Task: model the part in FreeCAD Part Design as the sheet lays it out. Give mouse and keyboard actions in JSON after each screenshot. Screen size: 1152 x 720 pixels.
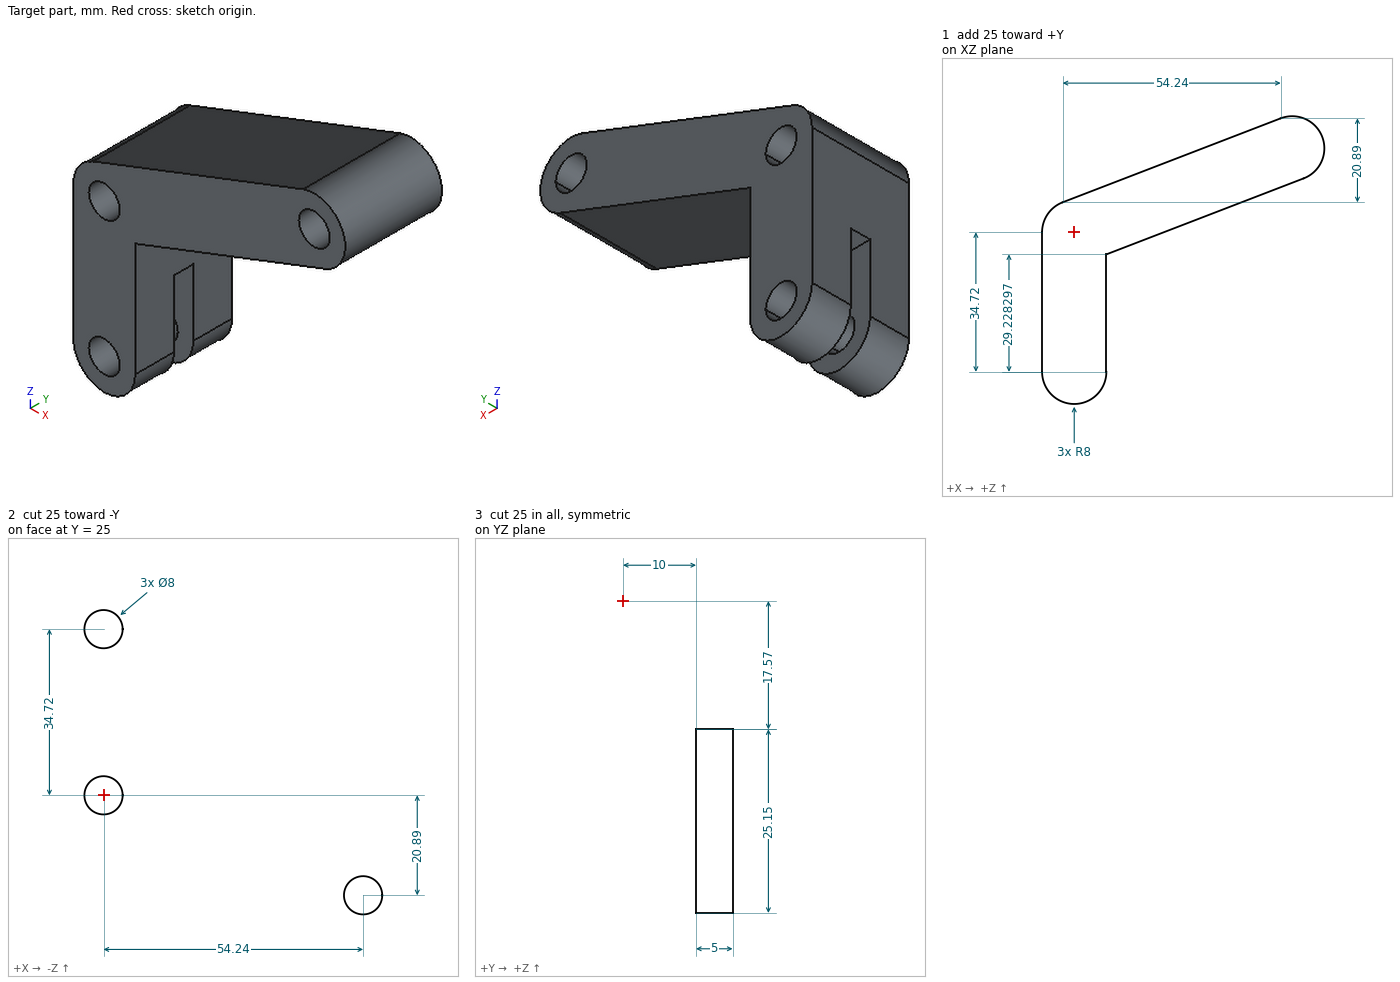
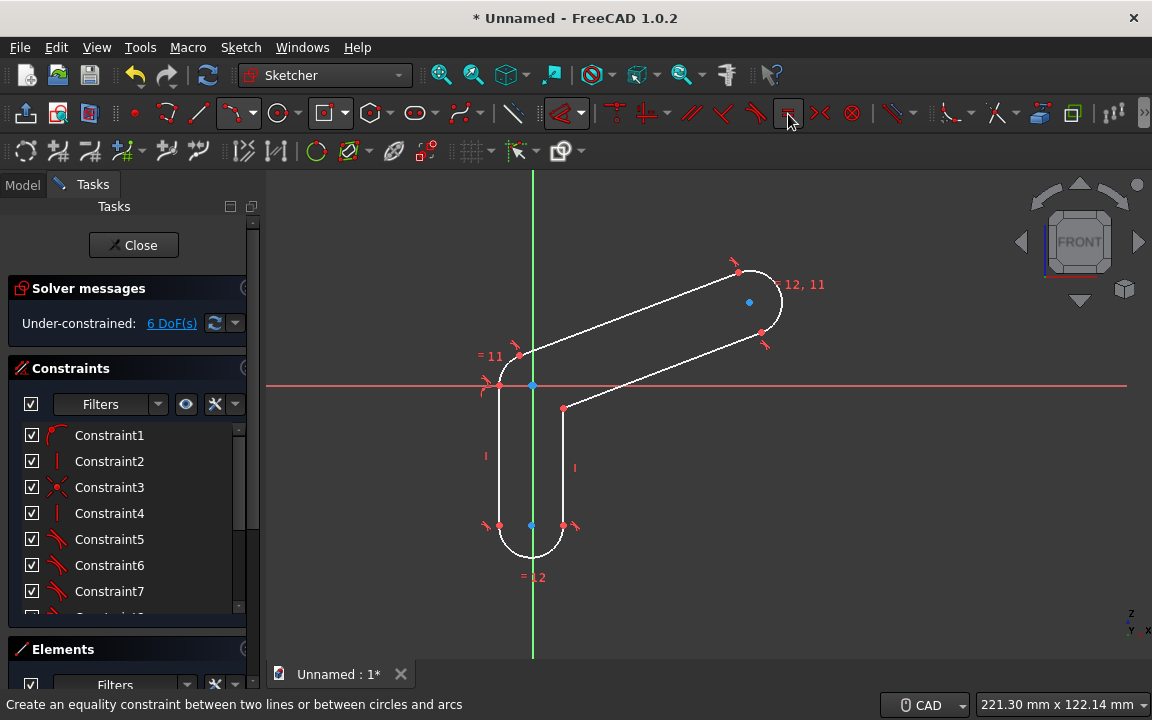
{"action": "left_click", "coordinate": [531, 386]}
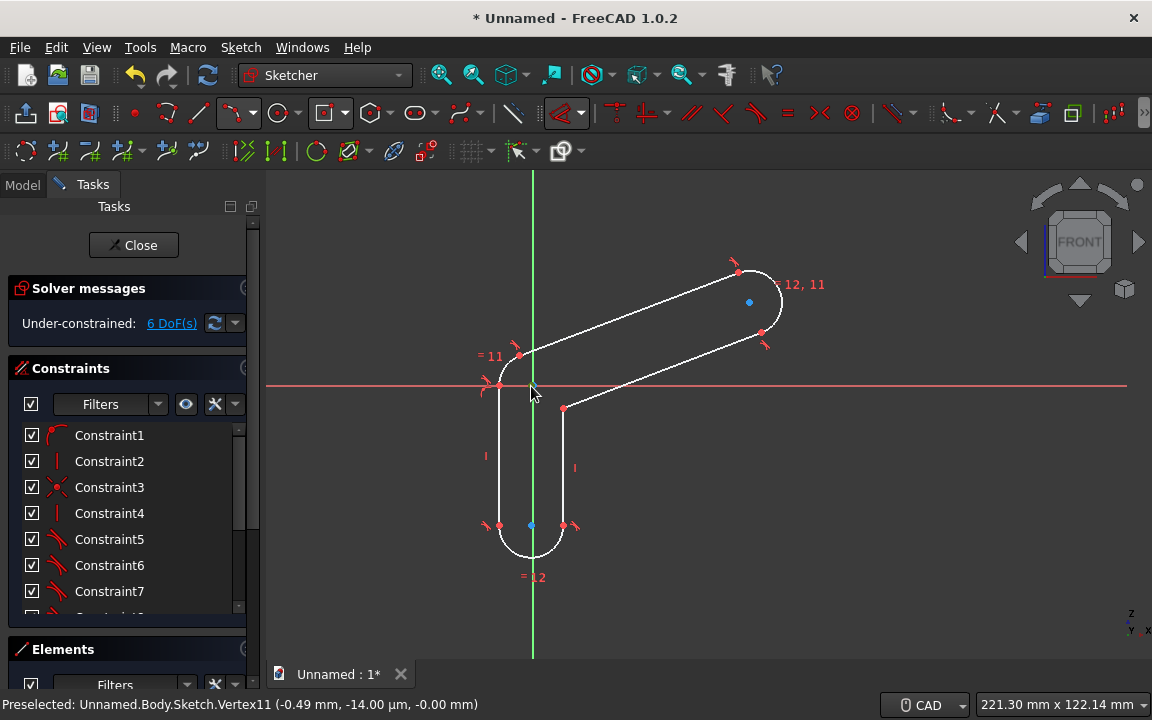
{"action": "left_click", "coordinate": [533, 600]}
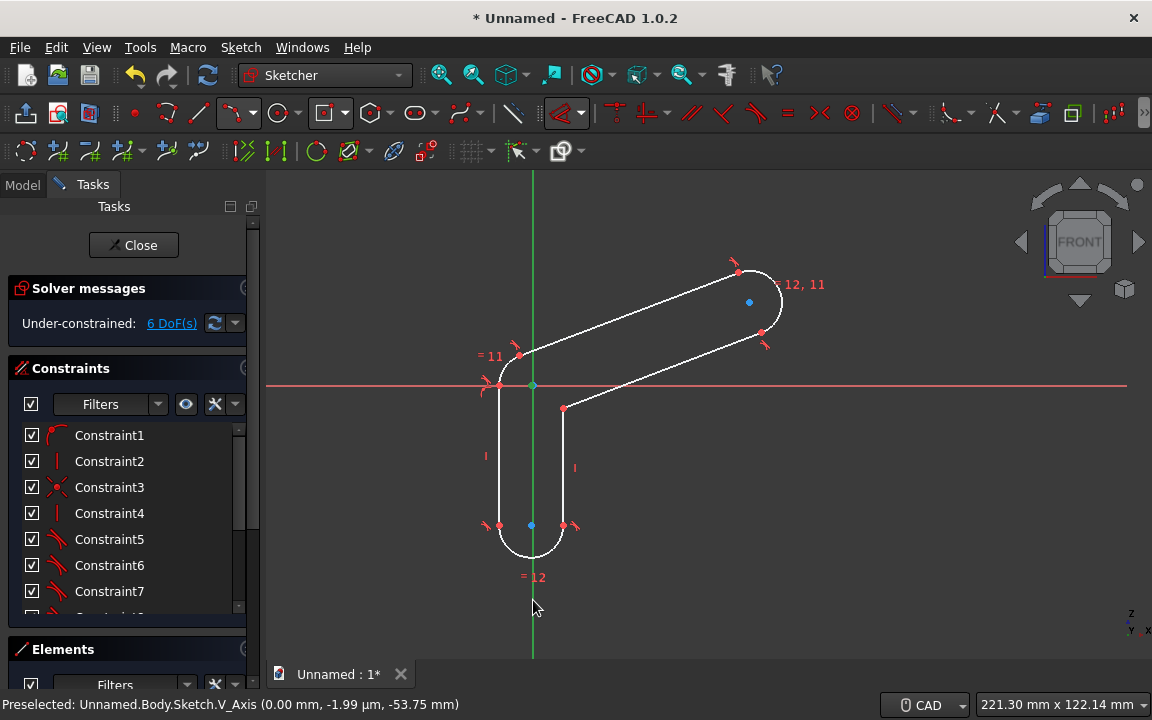
{"action": "left_click", "coordinate": [616, 114]}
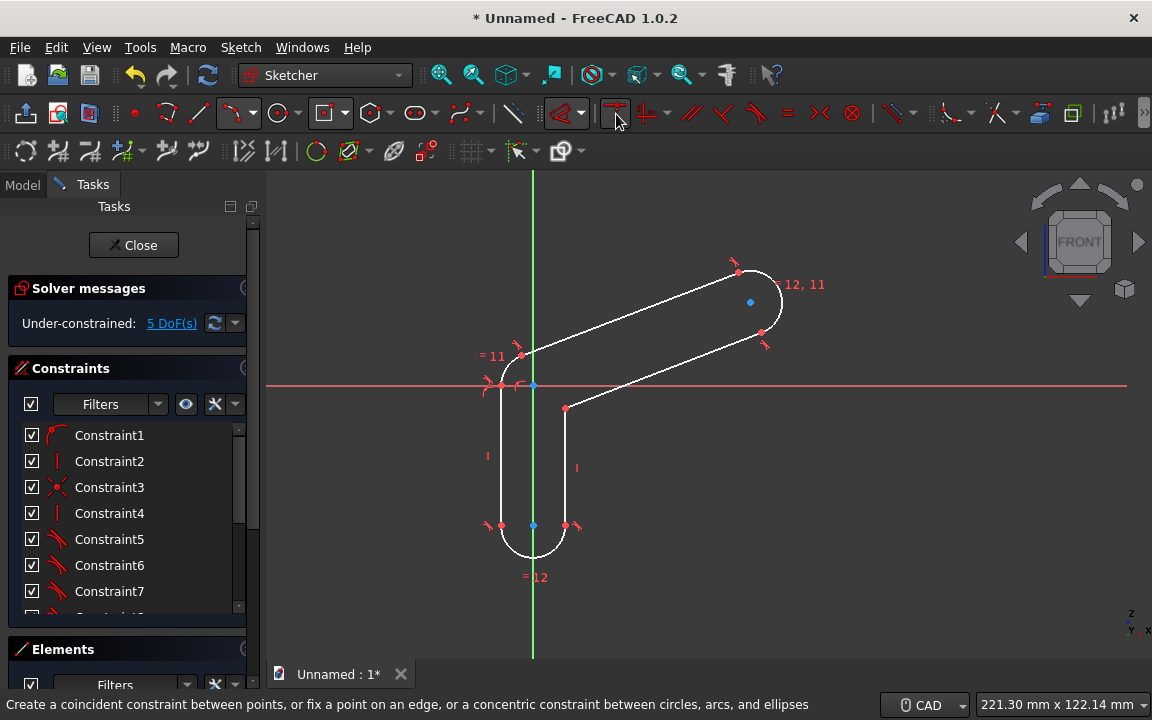
{"action": "scroll", "coordinate": [512, 362], "scroll_direction": "up", "scroll_amount": 2}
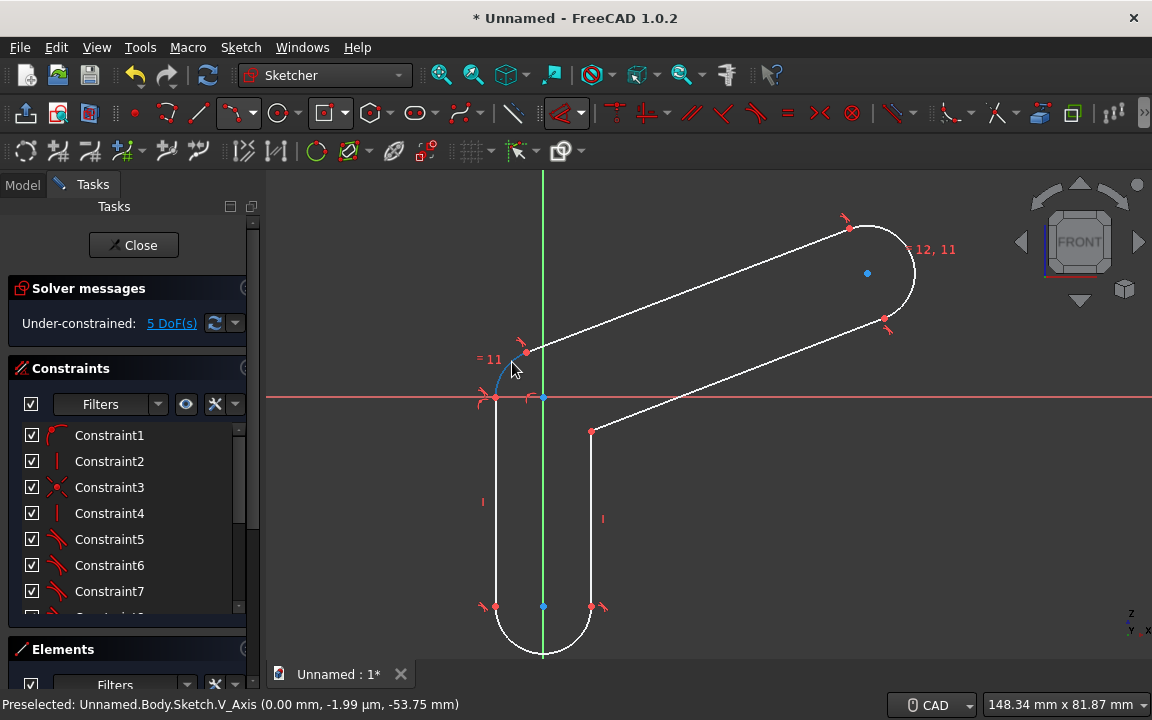
{"action": "left_click", "coordinate": [512, 362]}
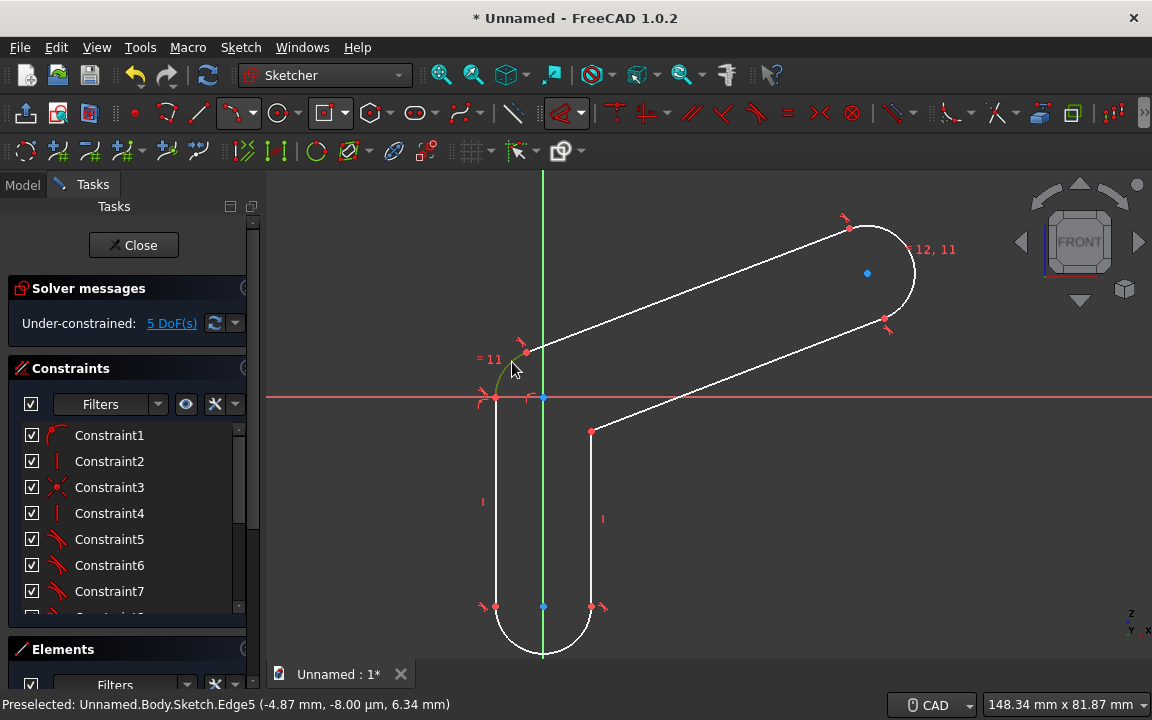
{"action": "key", "text": "k r"}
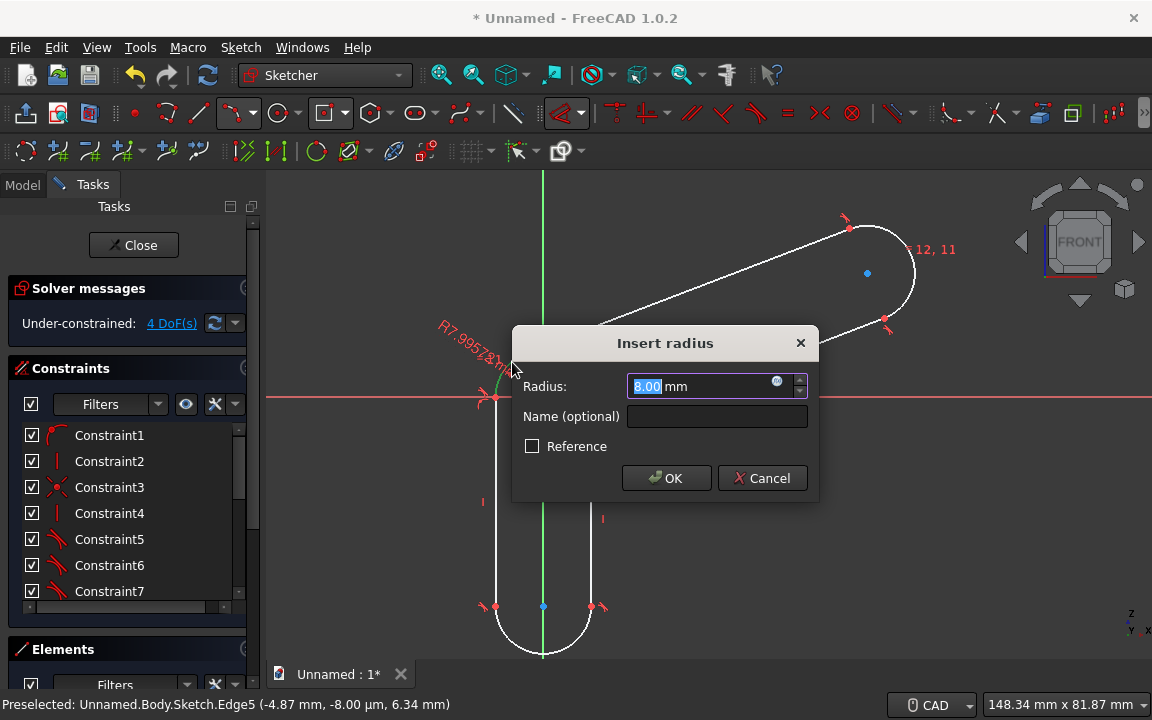
{"action": "type", "text": "8"}
{"action": "key", "text": "Return"}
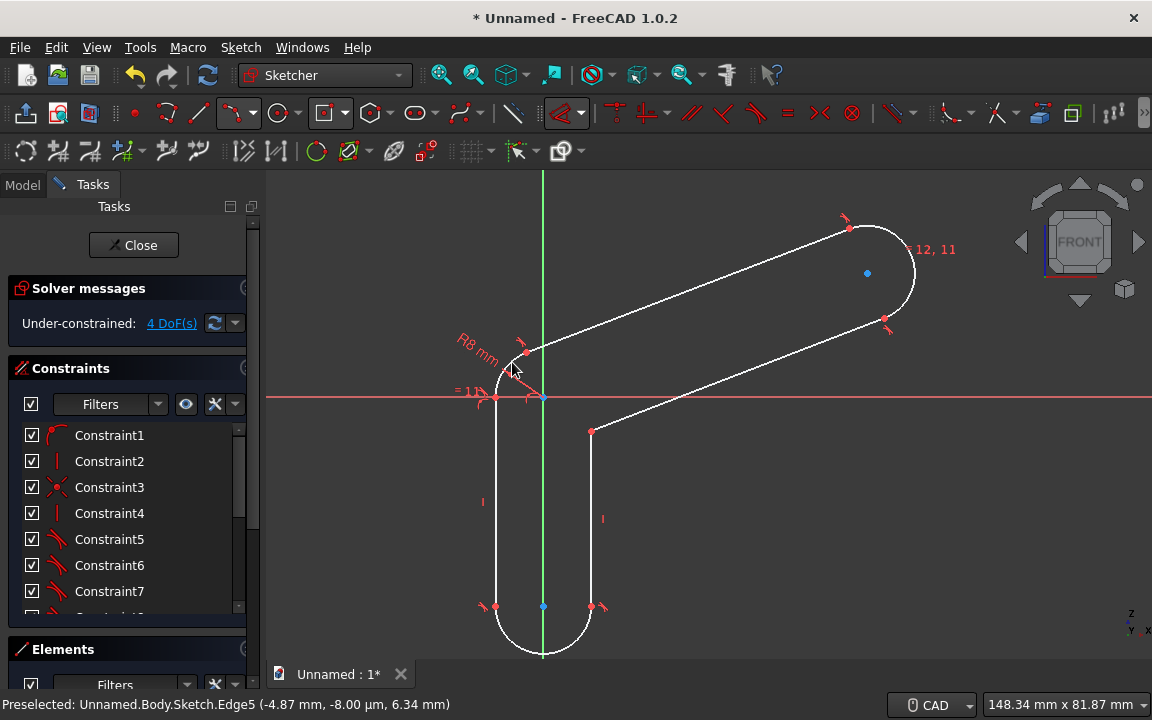
{"action": "left_click", "coordinate": [496, 543]}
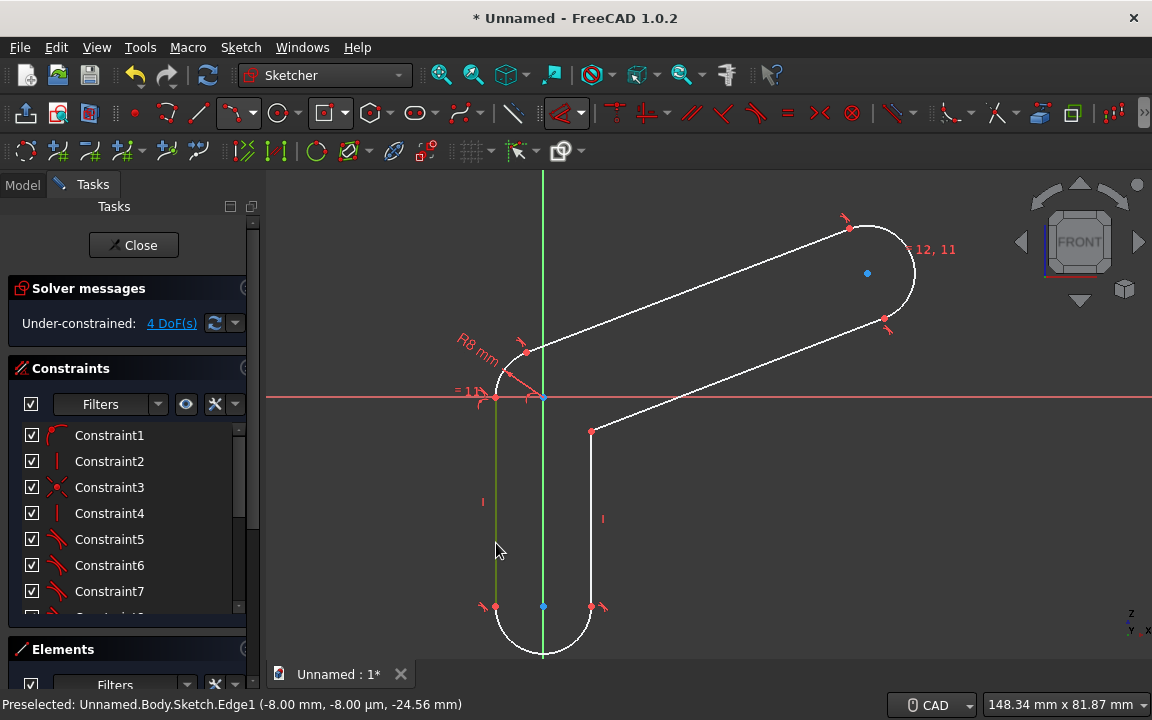
{"action": "key", "text": "i"}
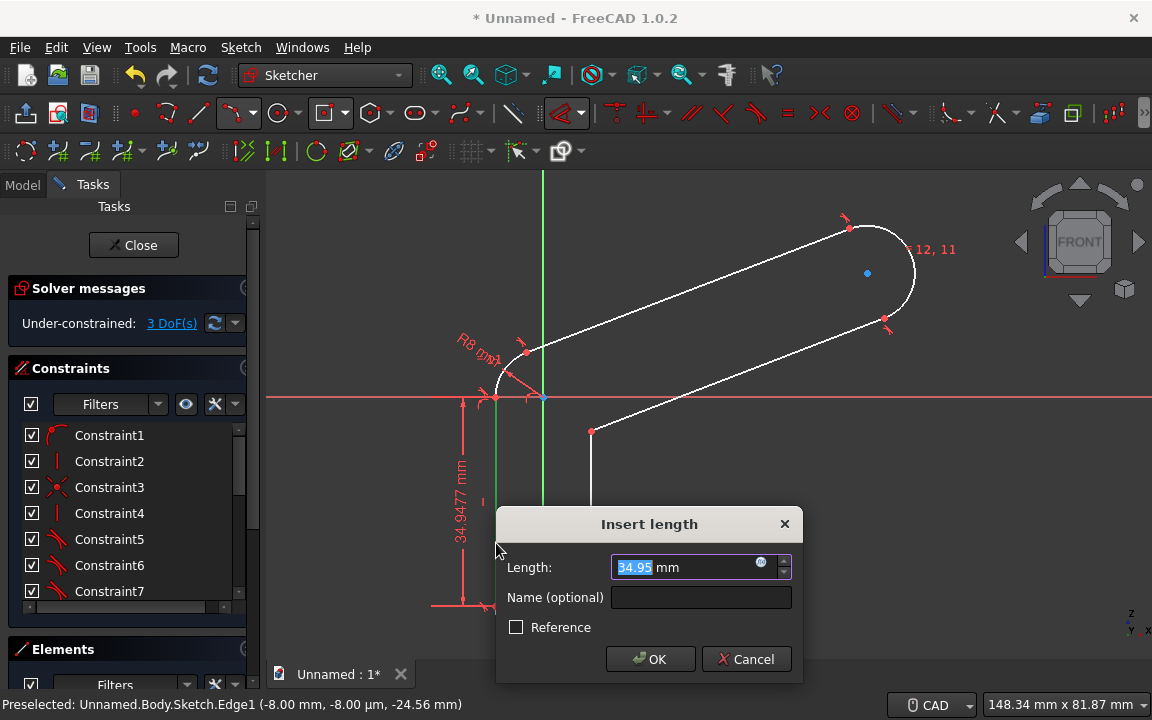
{"action": "type", "text": "34.72"}
{"action": "key", "text": "Return"}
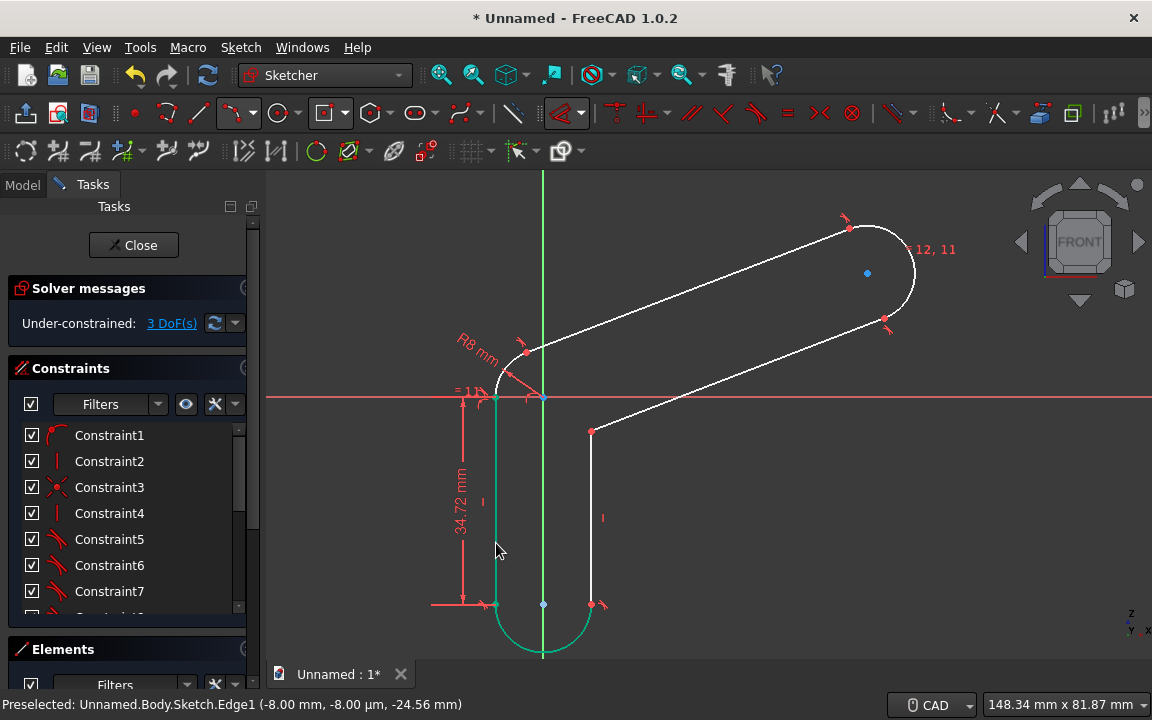
{"action": "left_click", "coordinate": [623, 316]}